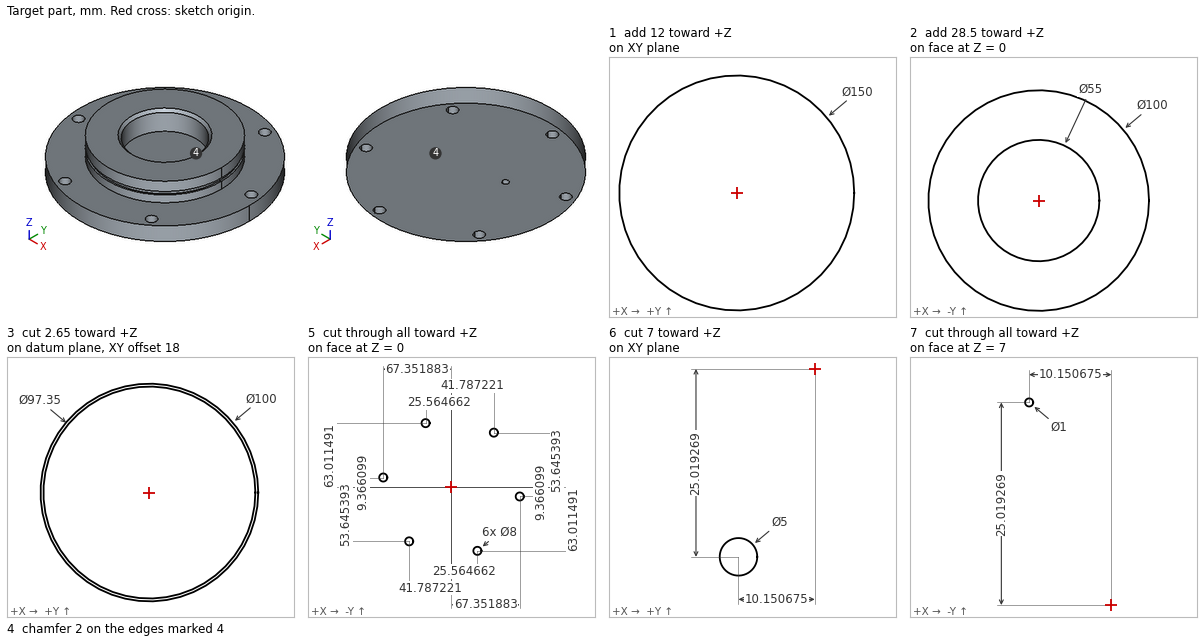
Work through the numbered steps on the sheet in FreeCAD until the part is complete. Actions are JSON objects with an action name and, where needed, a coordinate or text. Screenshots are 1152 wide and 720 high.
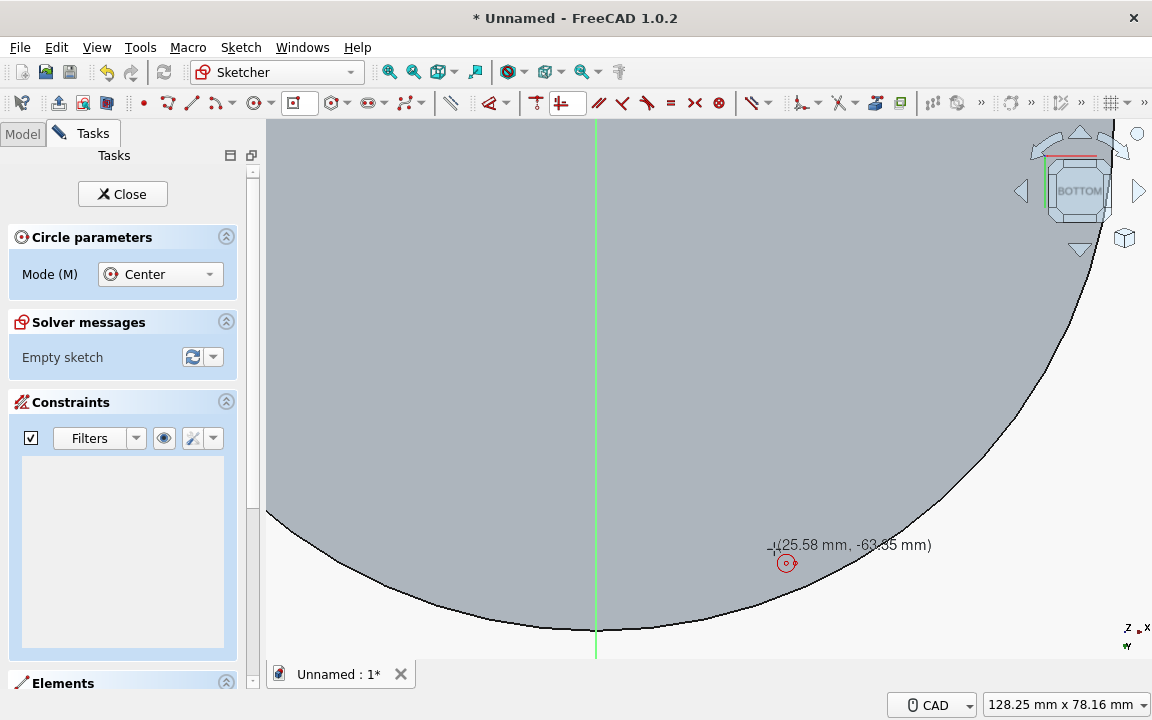
{"action": "left_click", "coordinate": [773, 548]}
{"action": "mouse_move", "coordinate": [792, 528]}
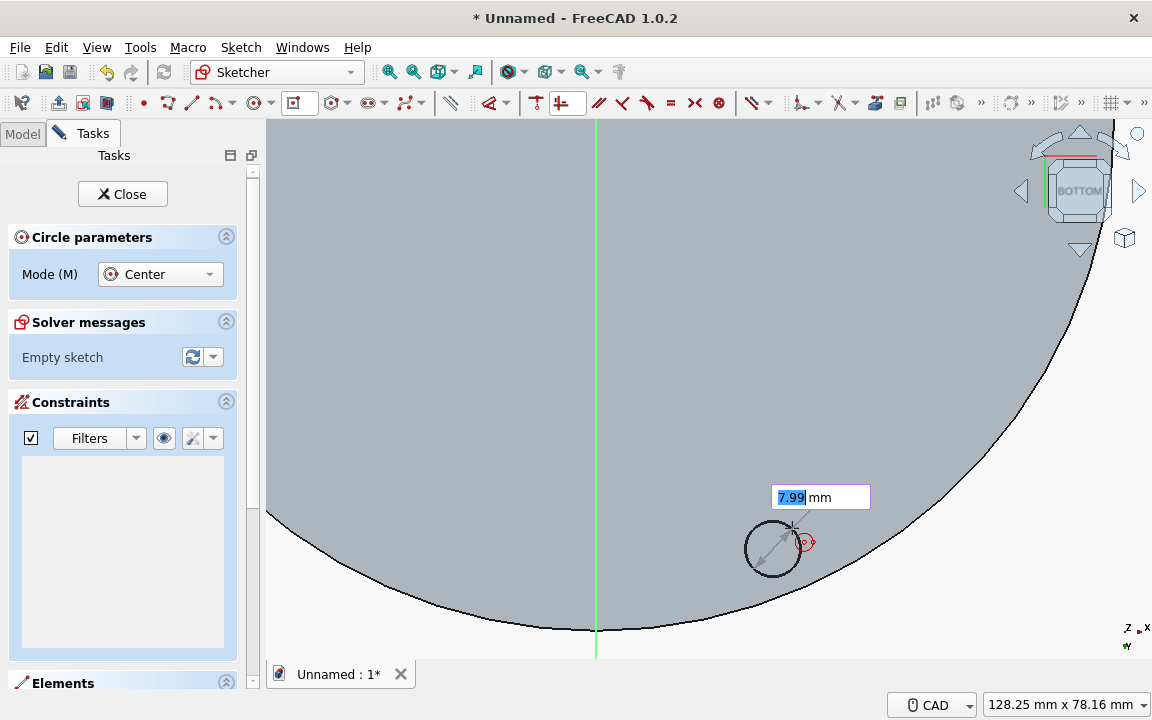
{"action": "type", "text": "8"}
{"action": "key", "text": "Return"}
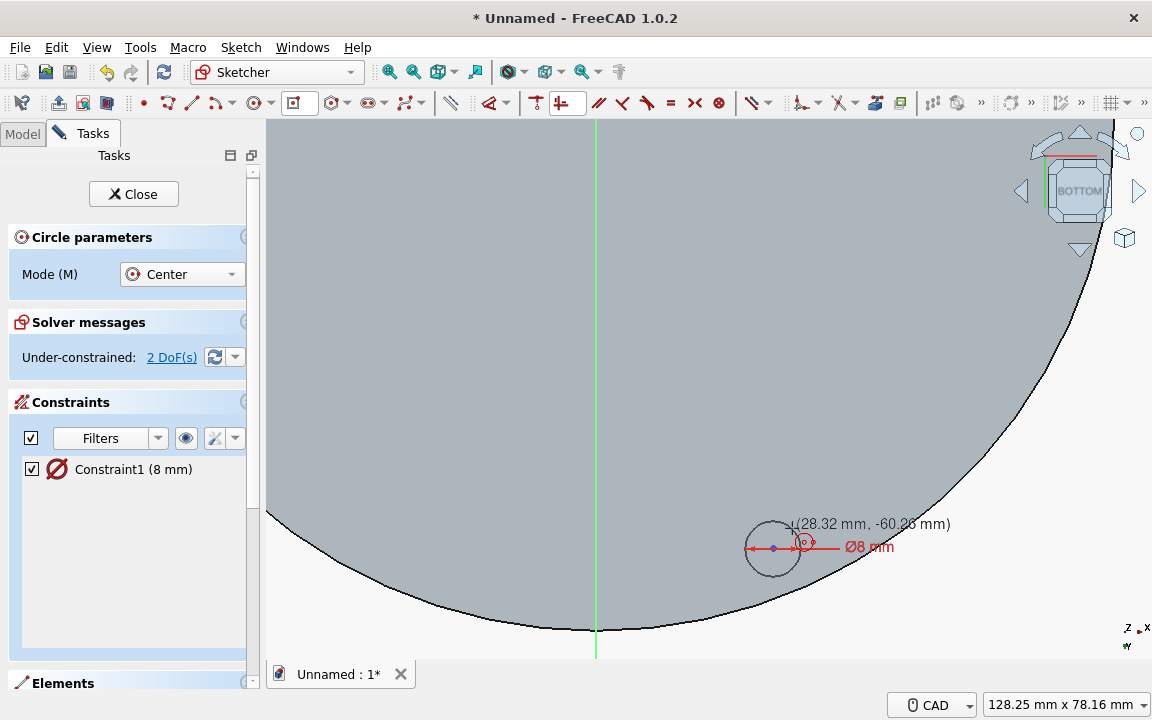
{"action": "left_click", "coordinate": [308, 483]}
{"action": "mouse_move", "coordinate": [327, 464]}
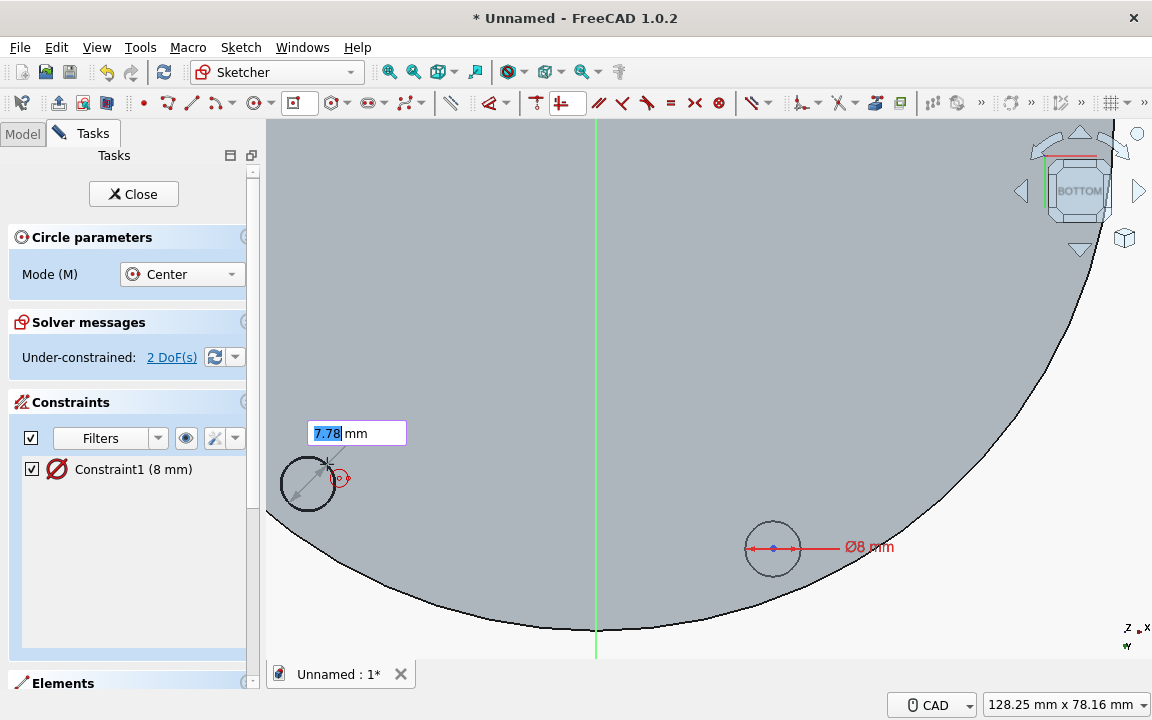
{"action": "type", "text": "8"}
{"action": "key", "text": "Return"}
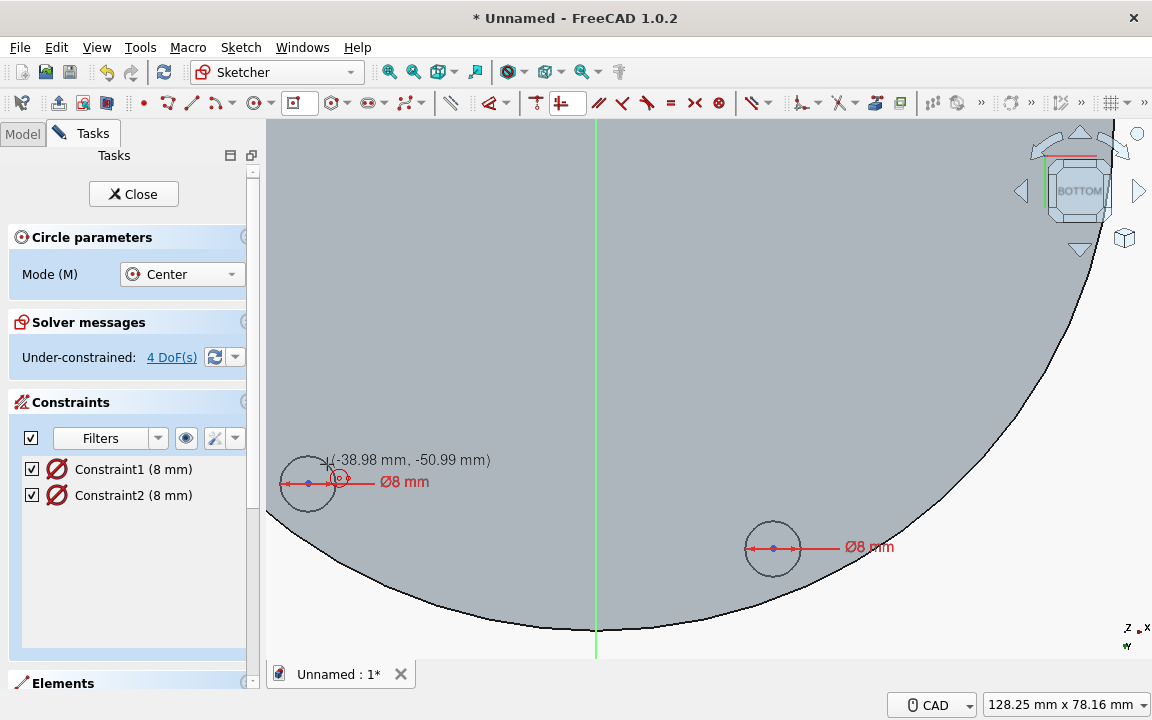
{"action": "scroll", "coordinate": [666, 550], "scroll_direction": "down", "scroll_amount": 5}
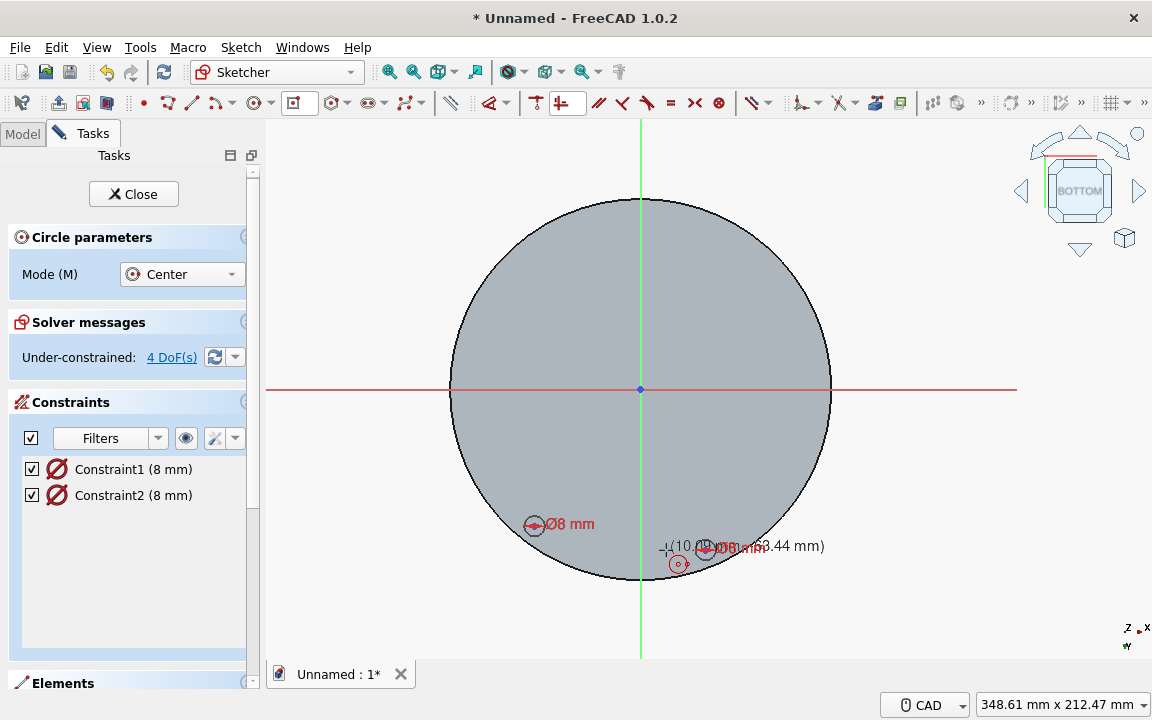
{"action": "scroll", "coordinate": [469, 366], "scroll_direction": "up", "scroll_amount": 5}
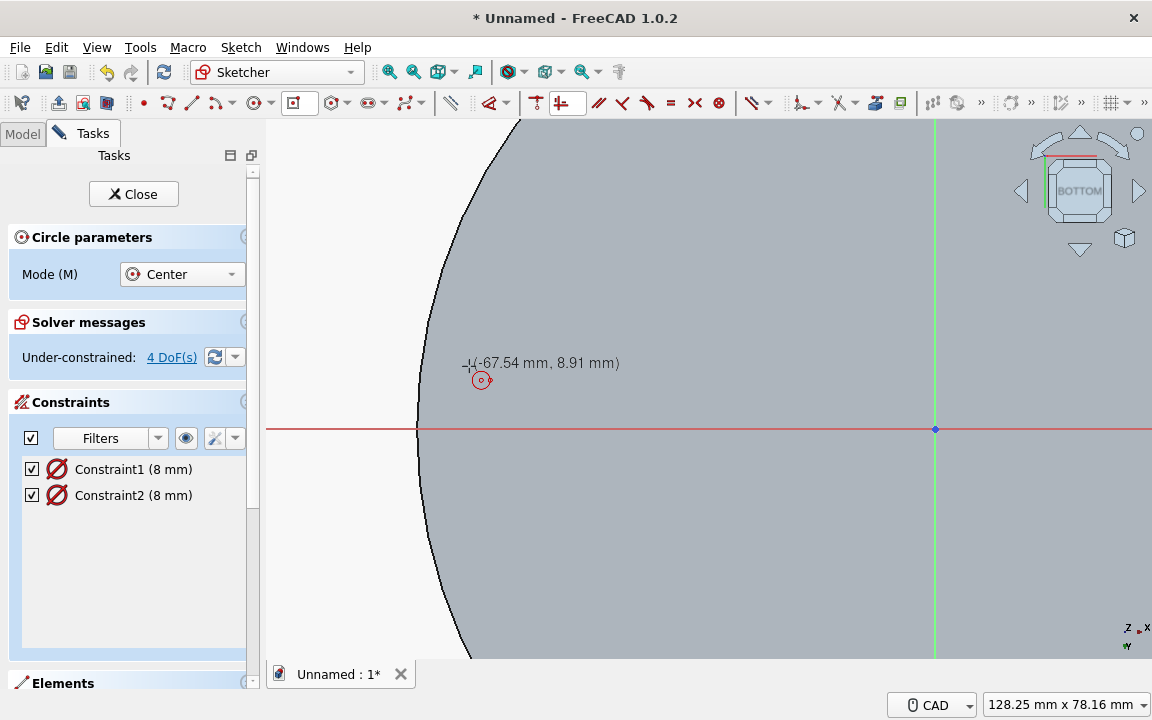
{"action": "left_click", "coordinate": [470, 365]}
{"action": "mouse_move", "coordinate": [489, 345]}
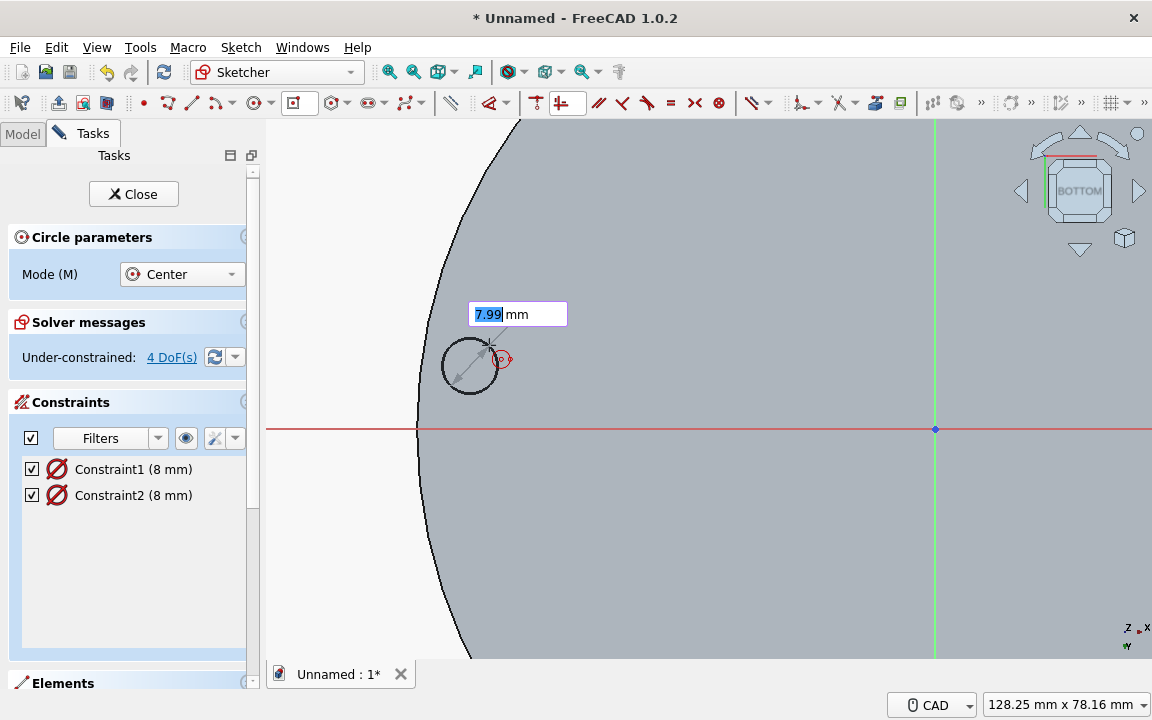
{"action": "type", "text": "8"}
{"action": "key", "text": "Return"}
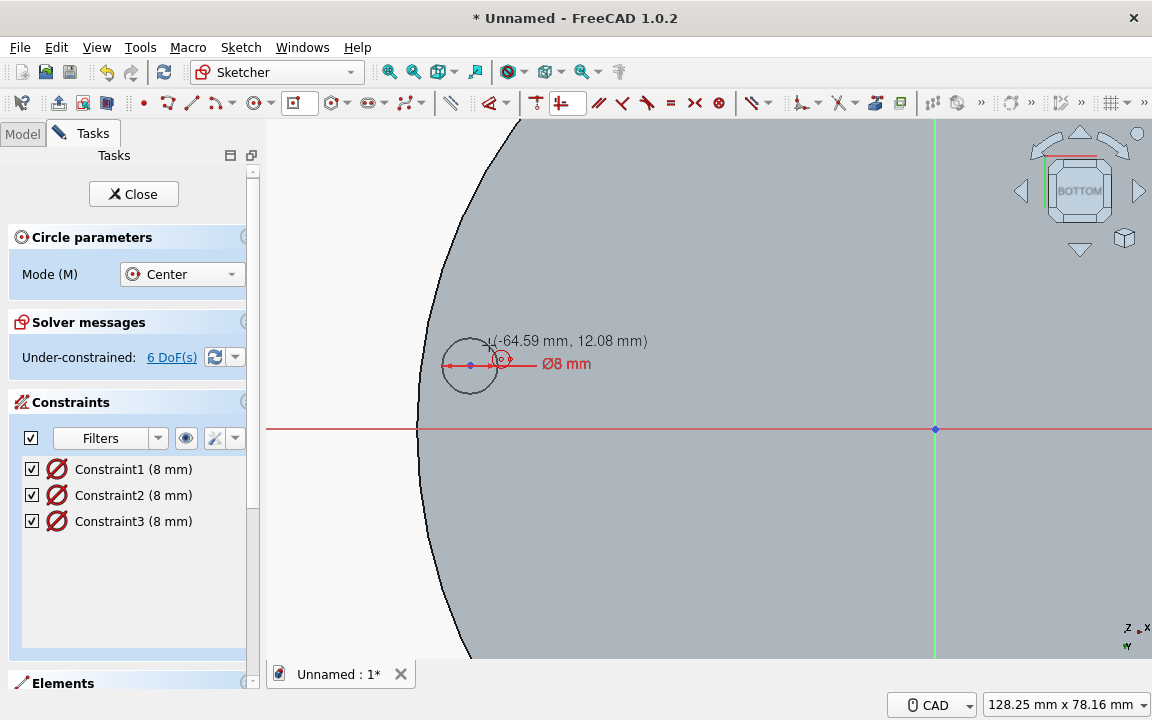
{"action": "scroll", "coordinate": [469, 365], "scroll_direction": "down", "scroll_amount": 5}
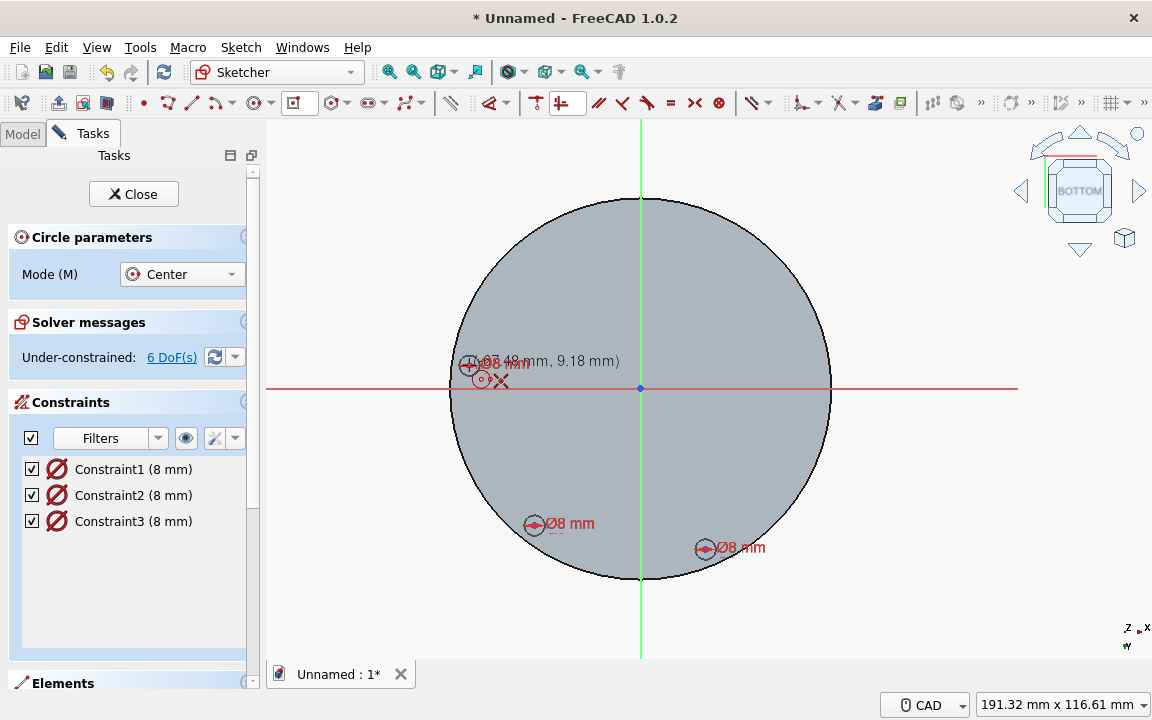
{"action": "scroll", "coordinate": [576, 229], "scroll_direction": "up", "scroll_amount": 5}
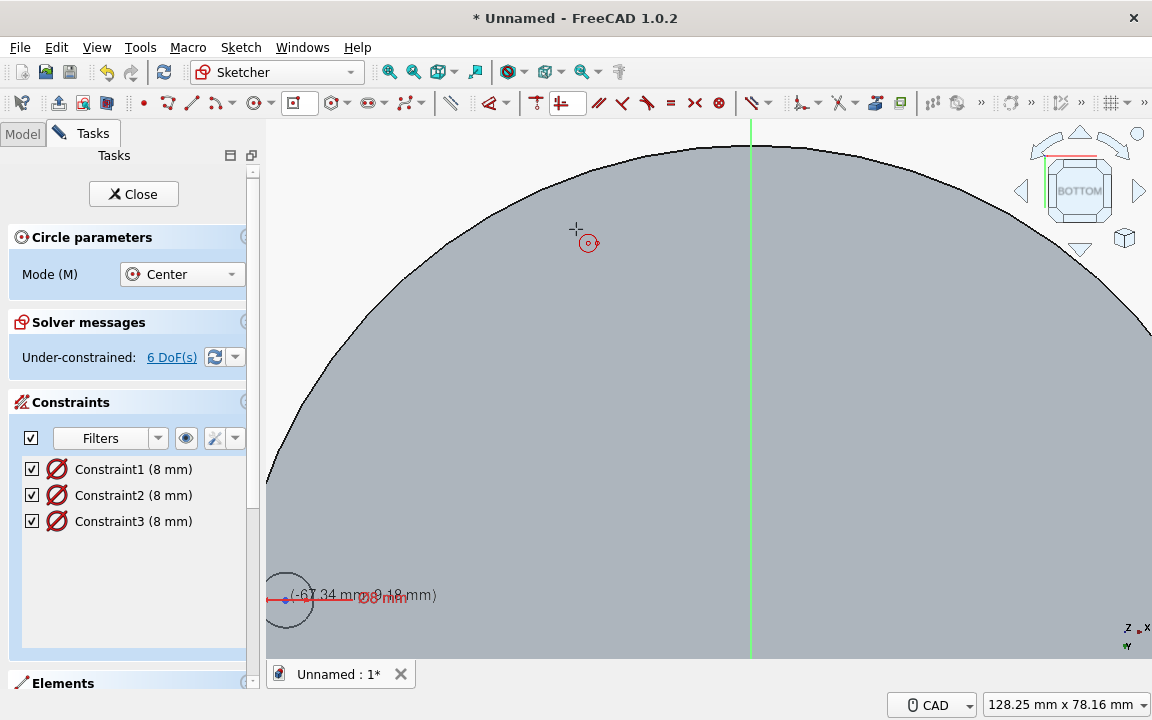
{"action": "left_click", "coordinate": [575, 228]}
{"action": "mouse_move", "coordinate": [594, 209]}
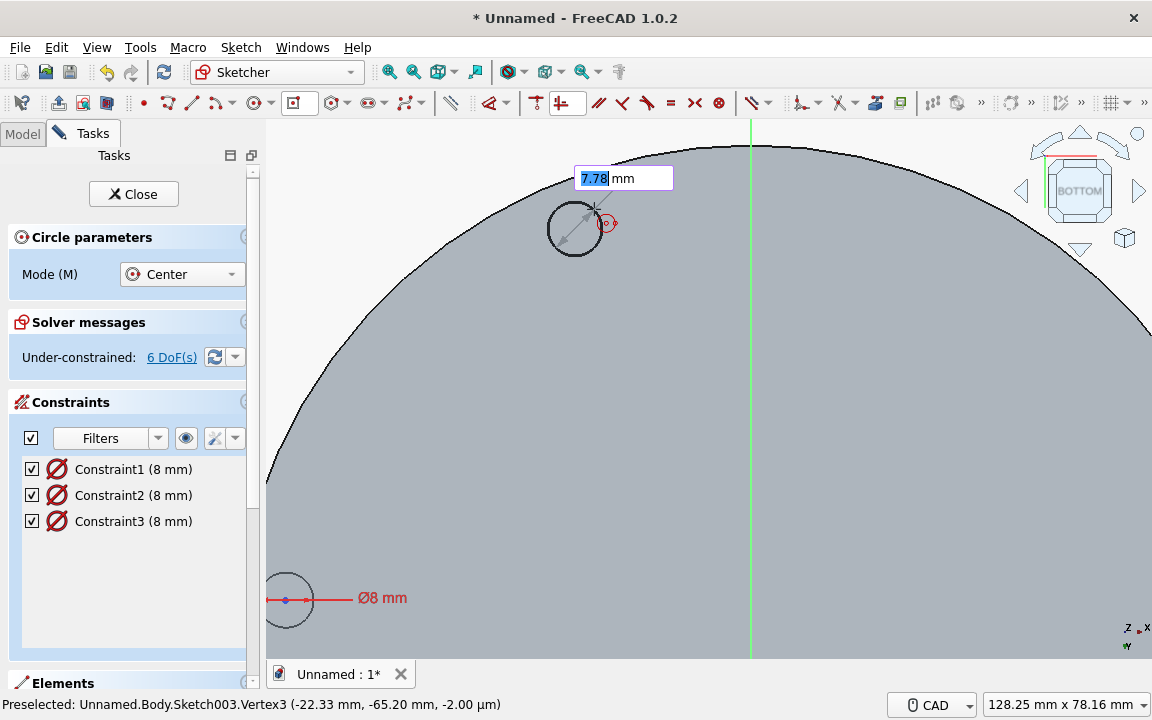
{"action": "type", "text": "8"}
{"action": "key", "text": "Return"}